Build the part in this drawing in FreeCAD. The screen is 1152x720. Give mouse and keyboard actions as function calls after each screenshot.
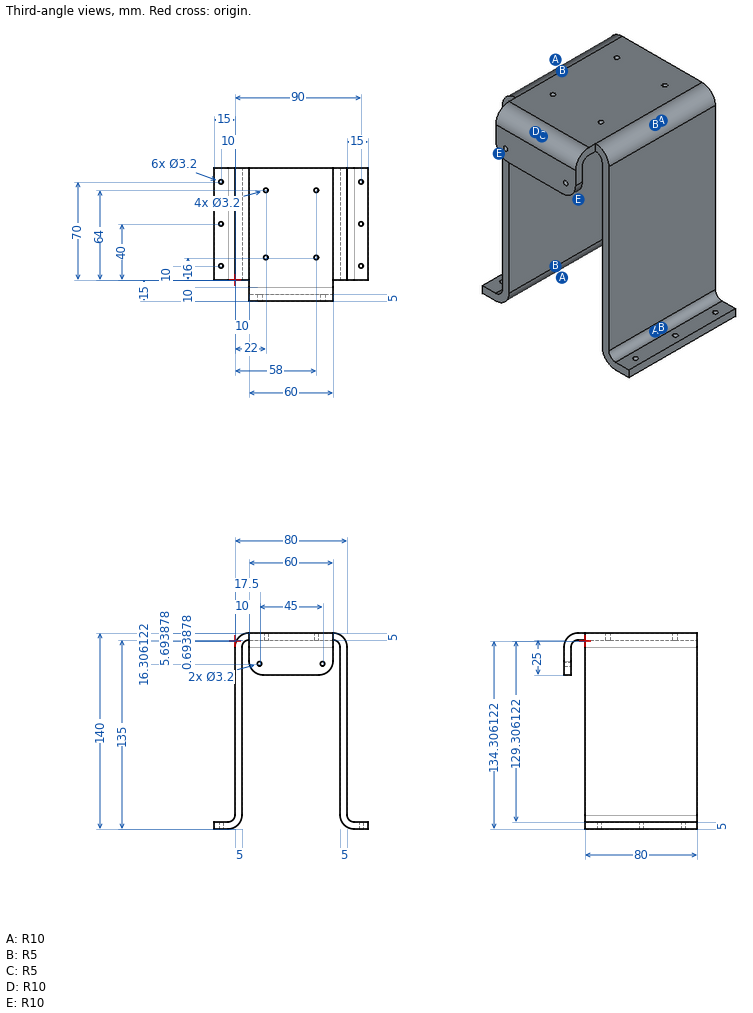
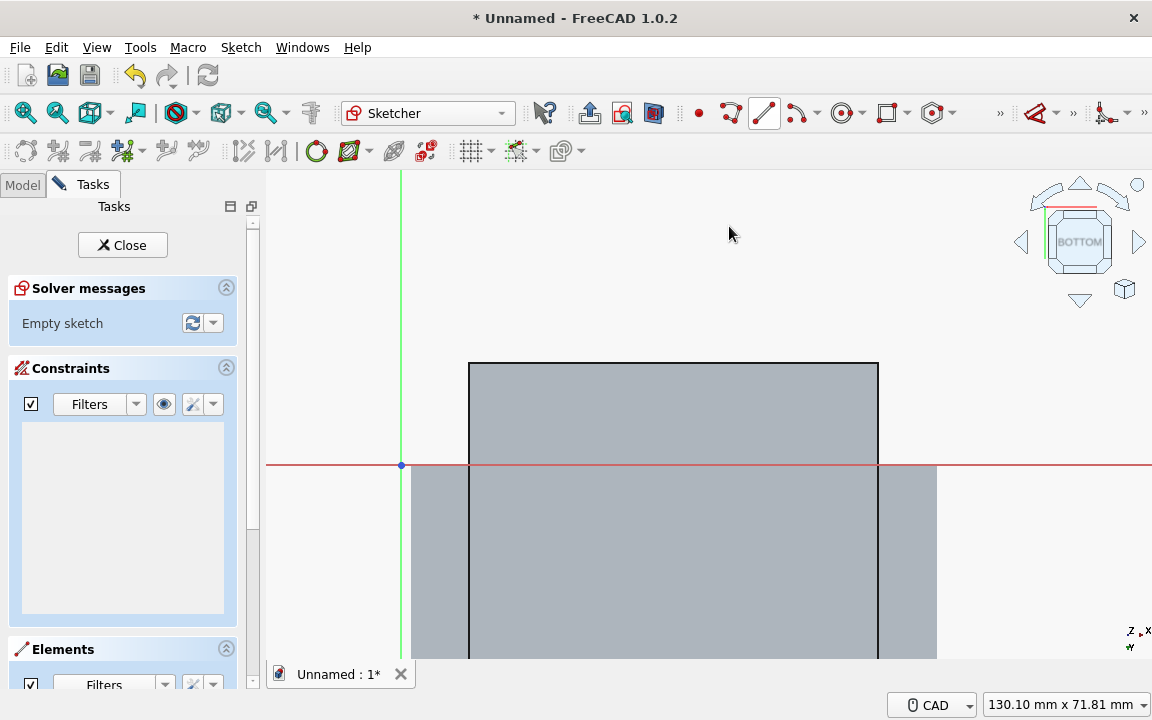
click(888, 114)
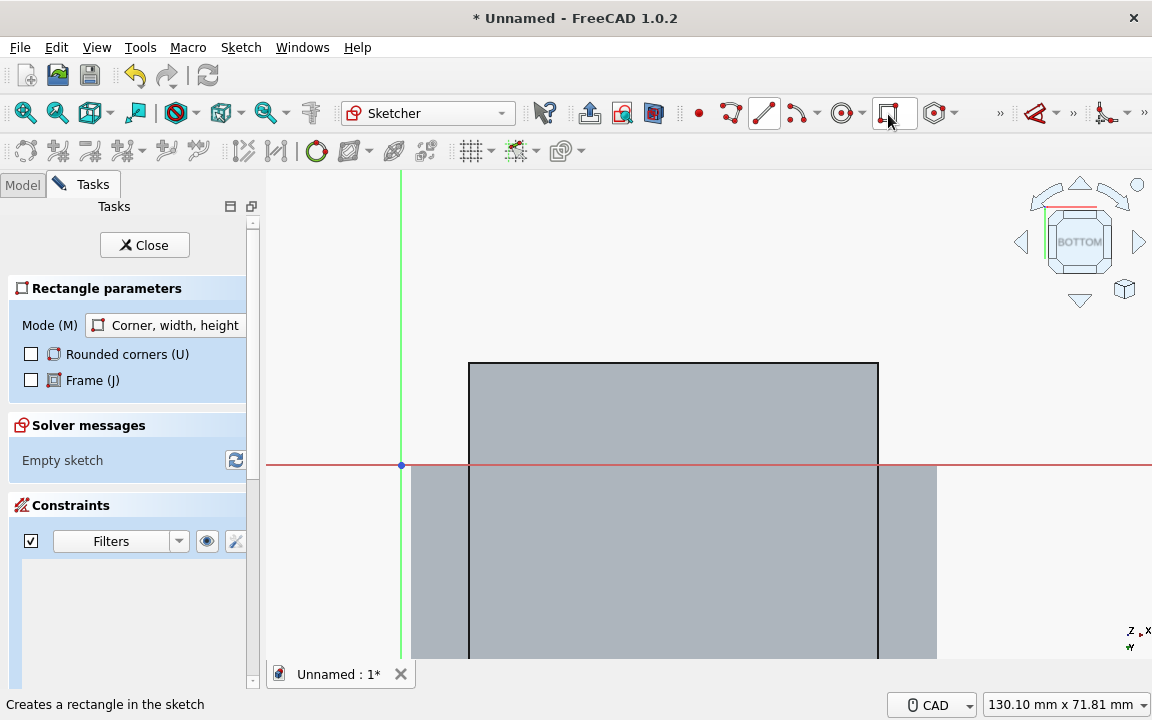
click(469, 363)
move(878, 397)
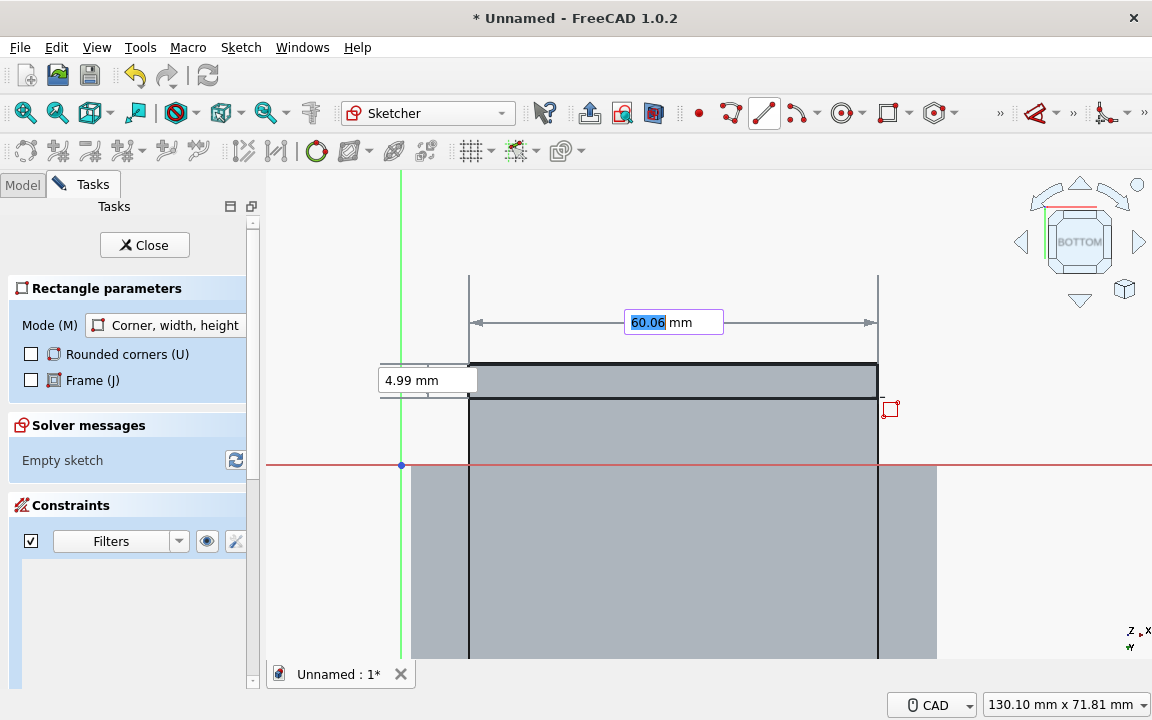
text(60)
key(Tab)
text(5)
key(Return)
key(Escape)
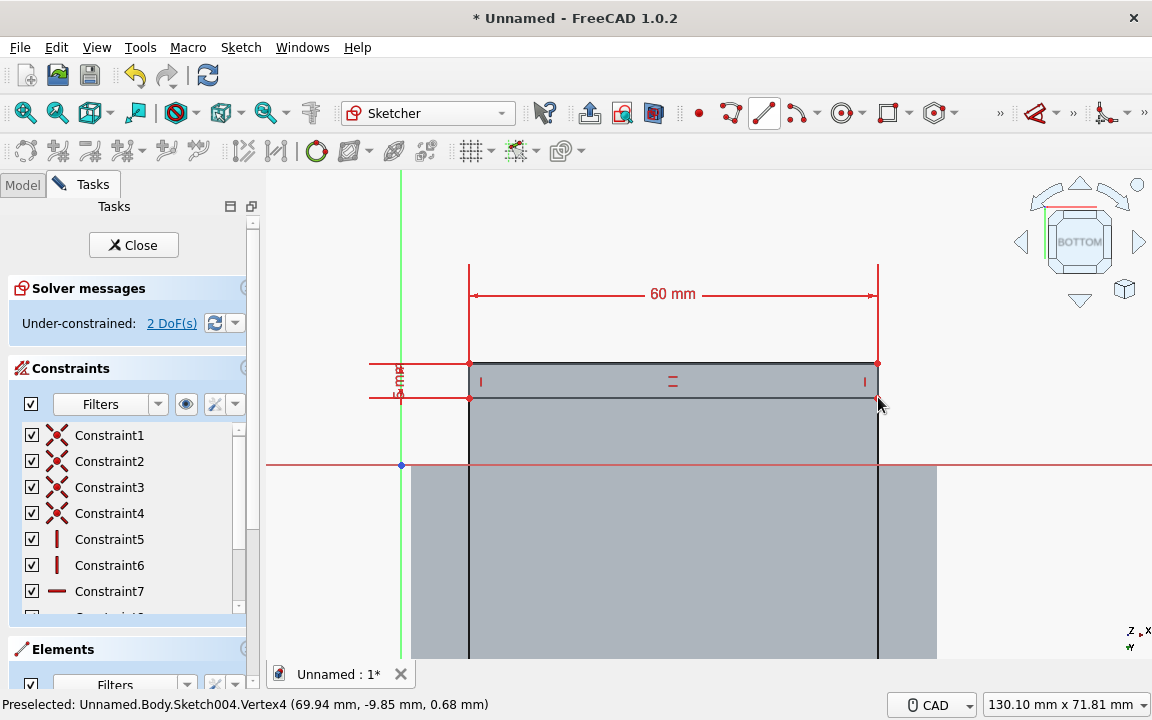
click(1036, 114)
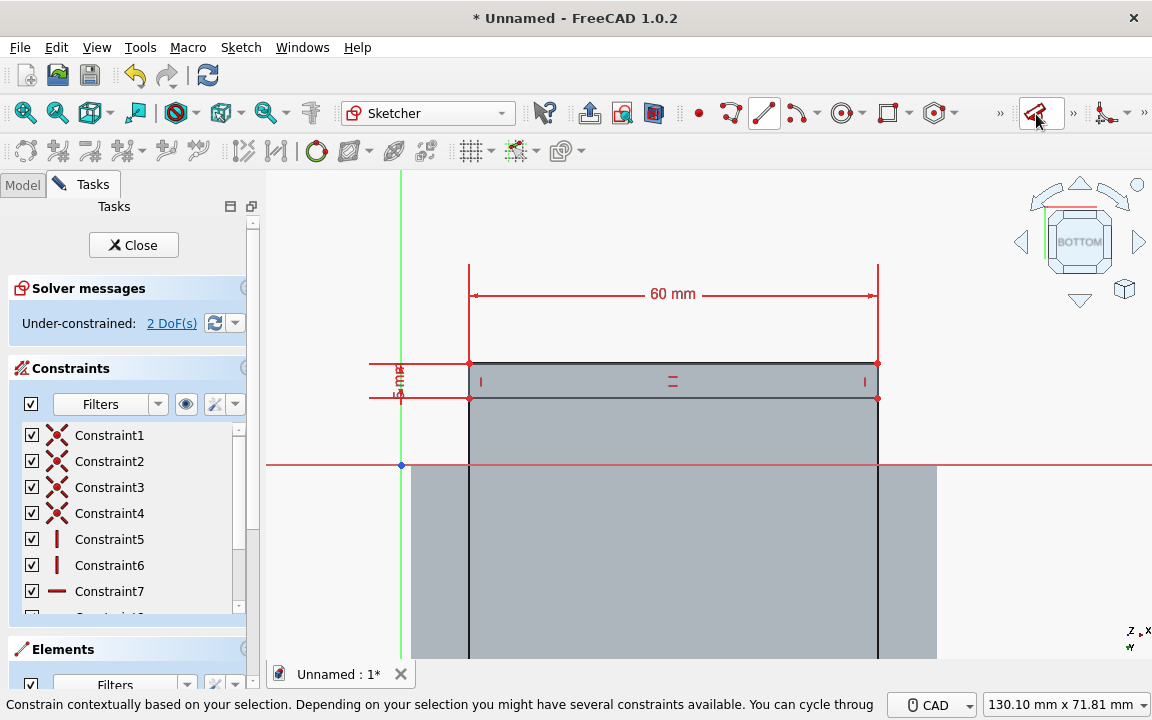
click(469, 364)
click(435, 499)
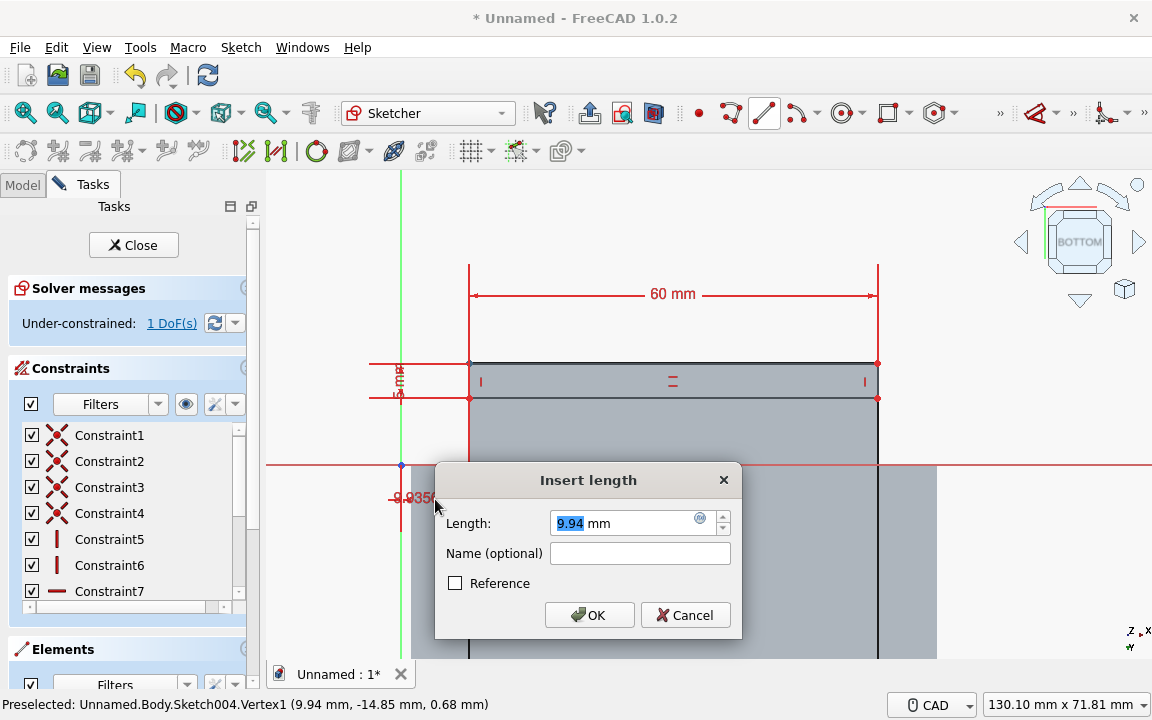
text(10)
key(Return)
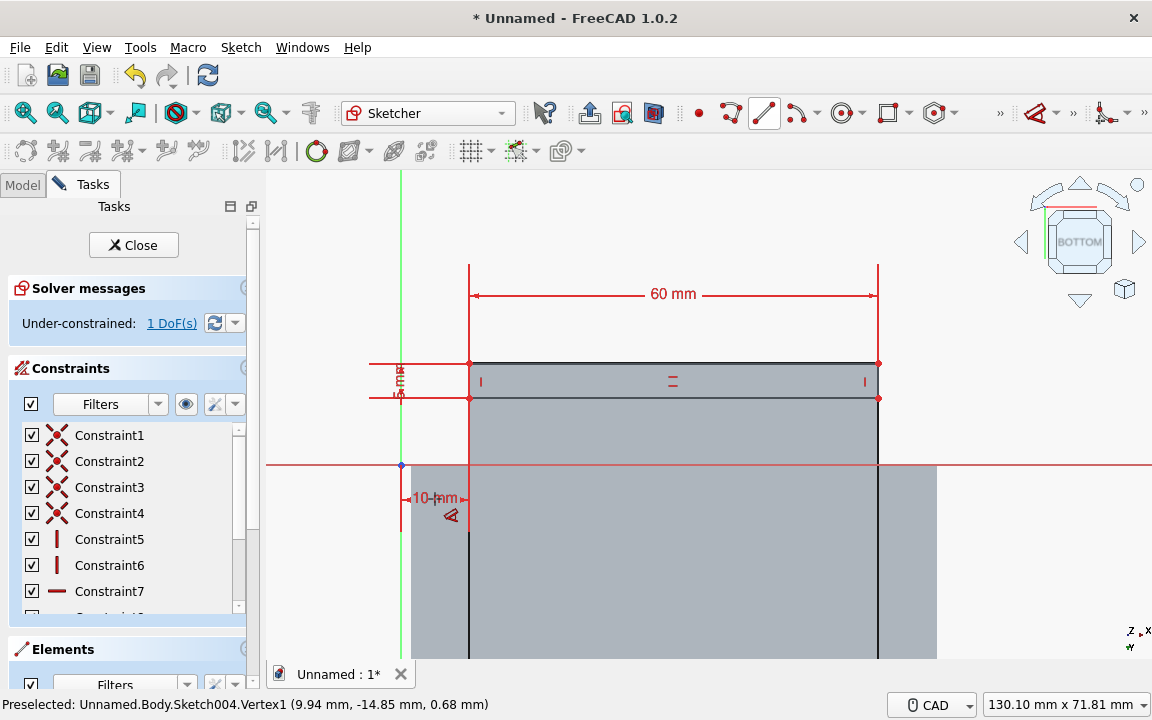
click(469, 364)
click(367, 415)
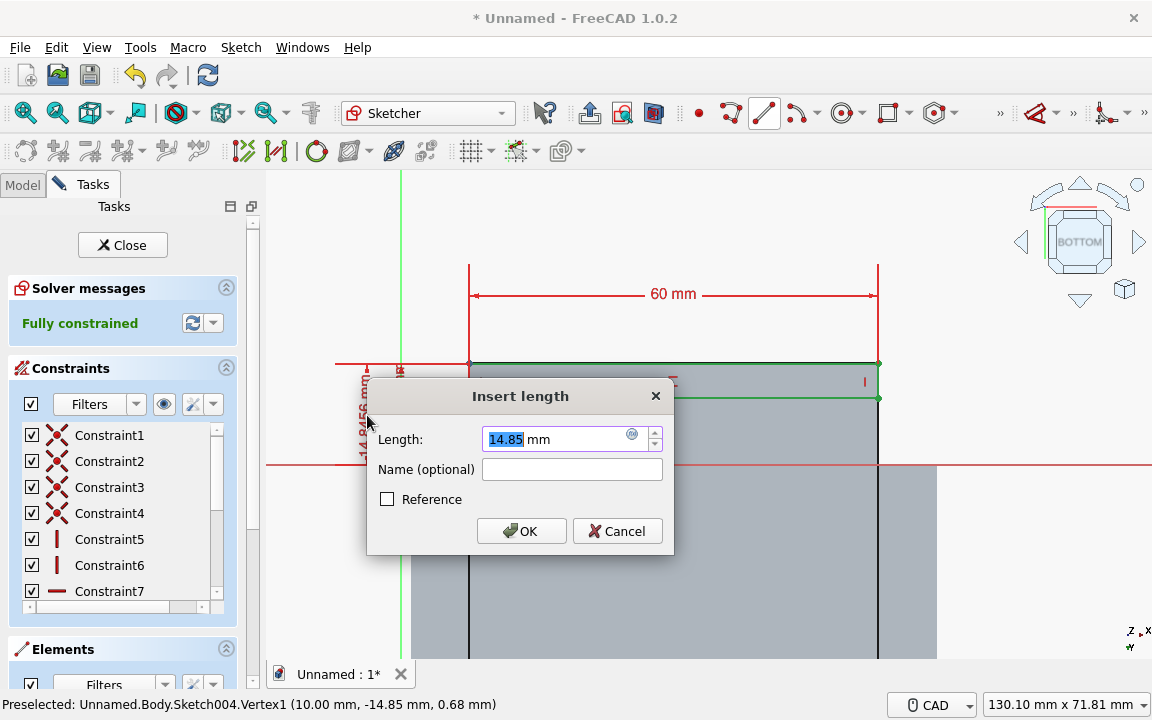
text(15)
key(Return)
key(Escape)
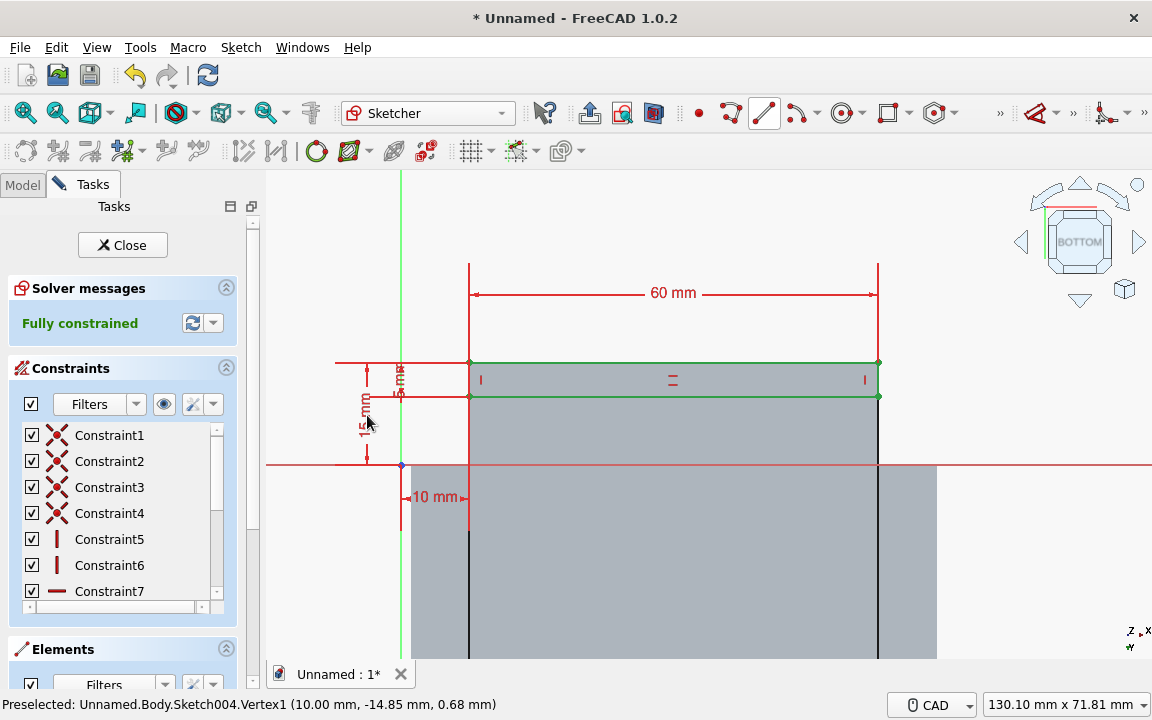
click(123, 245)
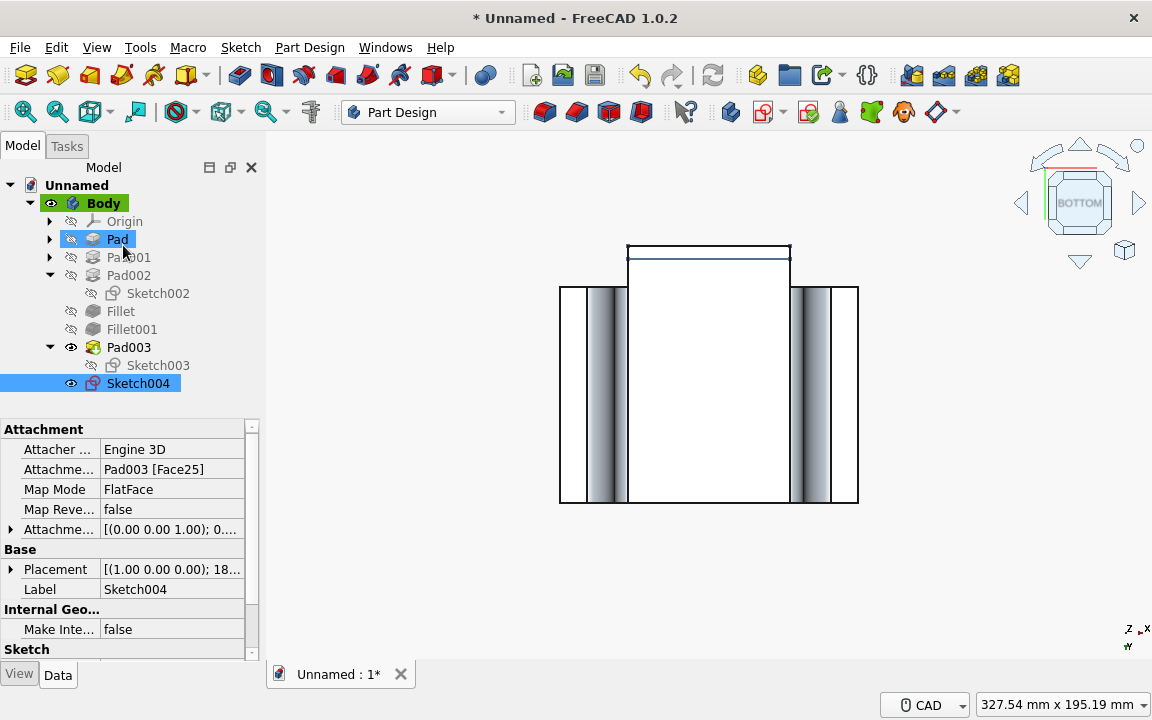
click(26, 76)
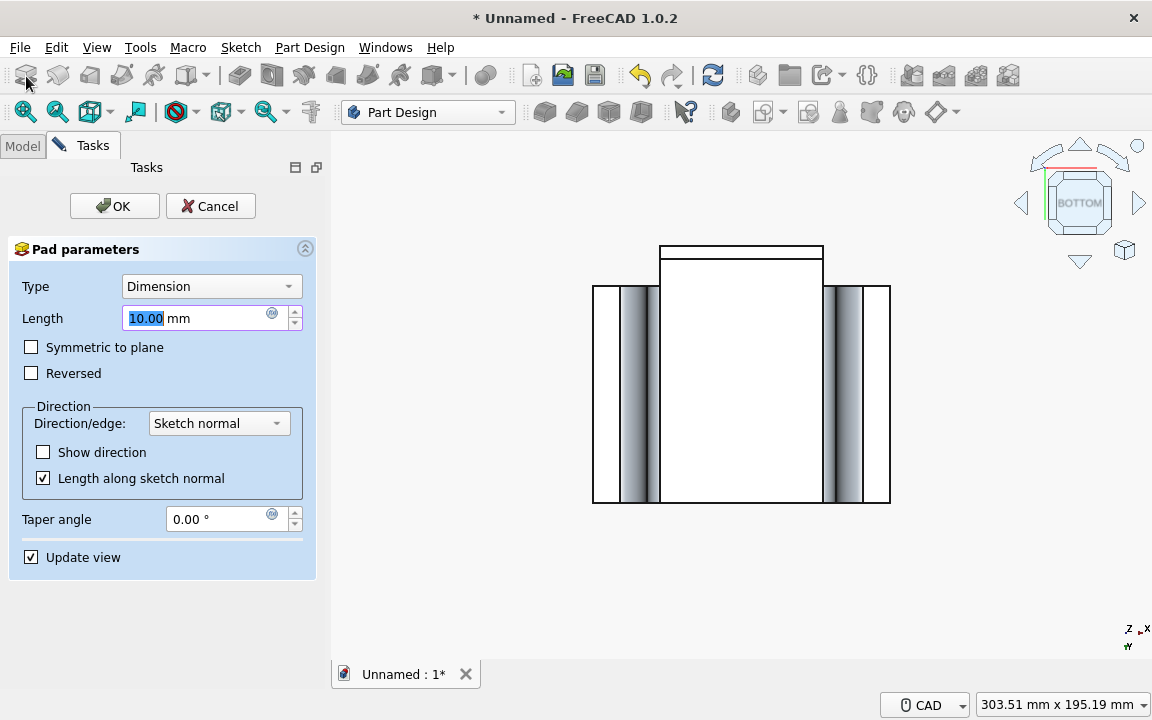
text(25)
key(Tab)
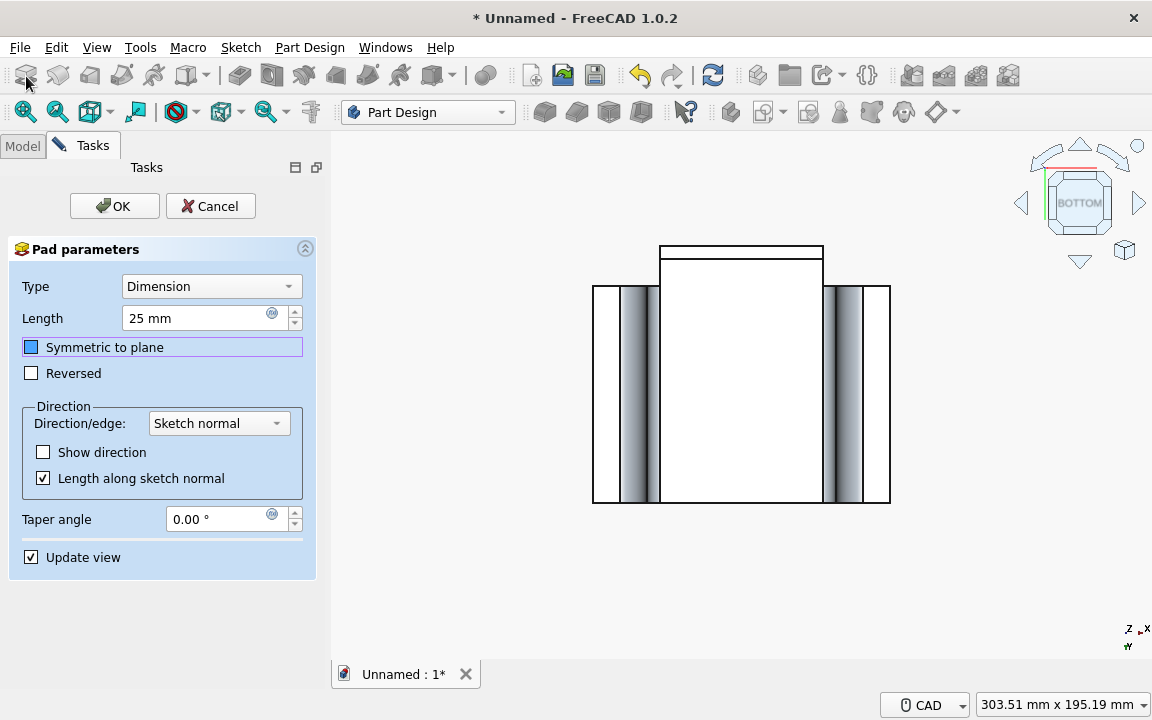
click(115, 206)